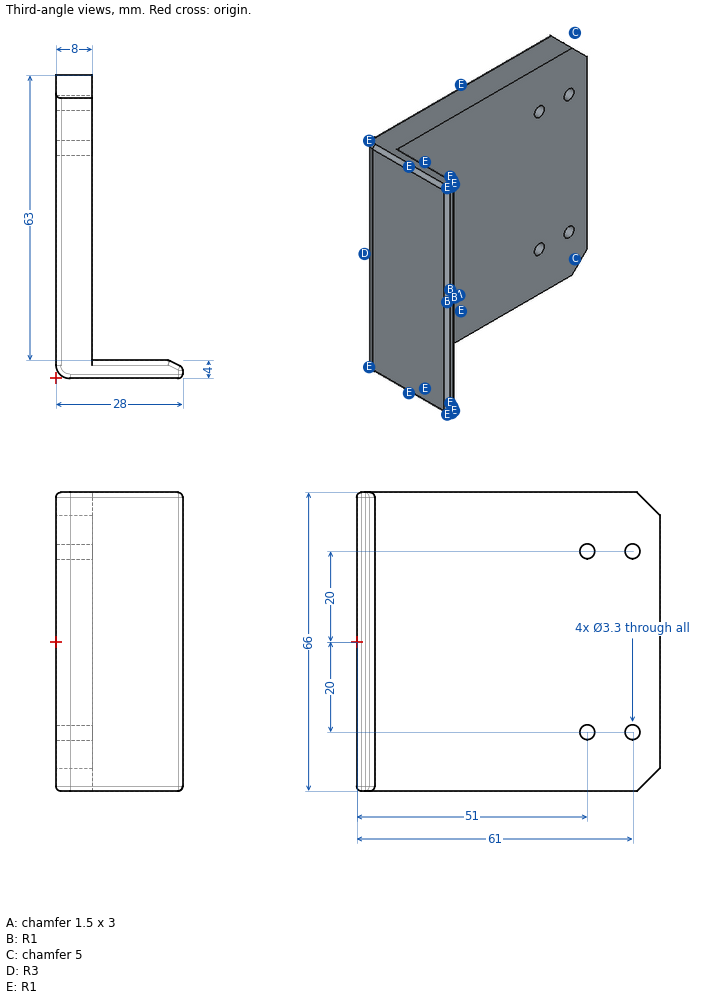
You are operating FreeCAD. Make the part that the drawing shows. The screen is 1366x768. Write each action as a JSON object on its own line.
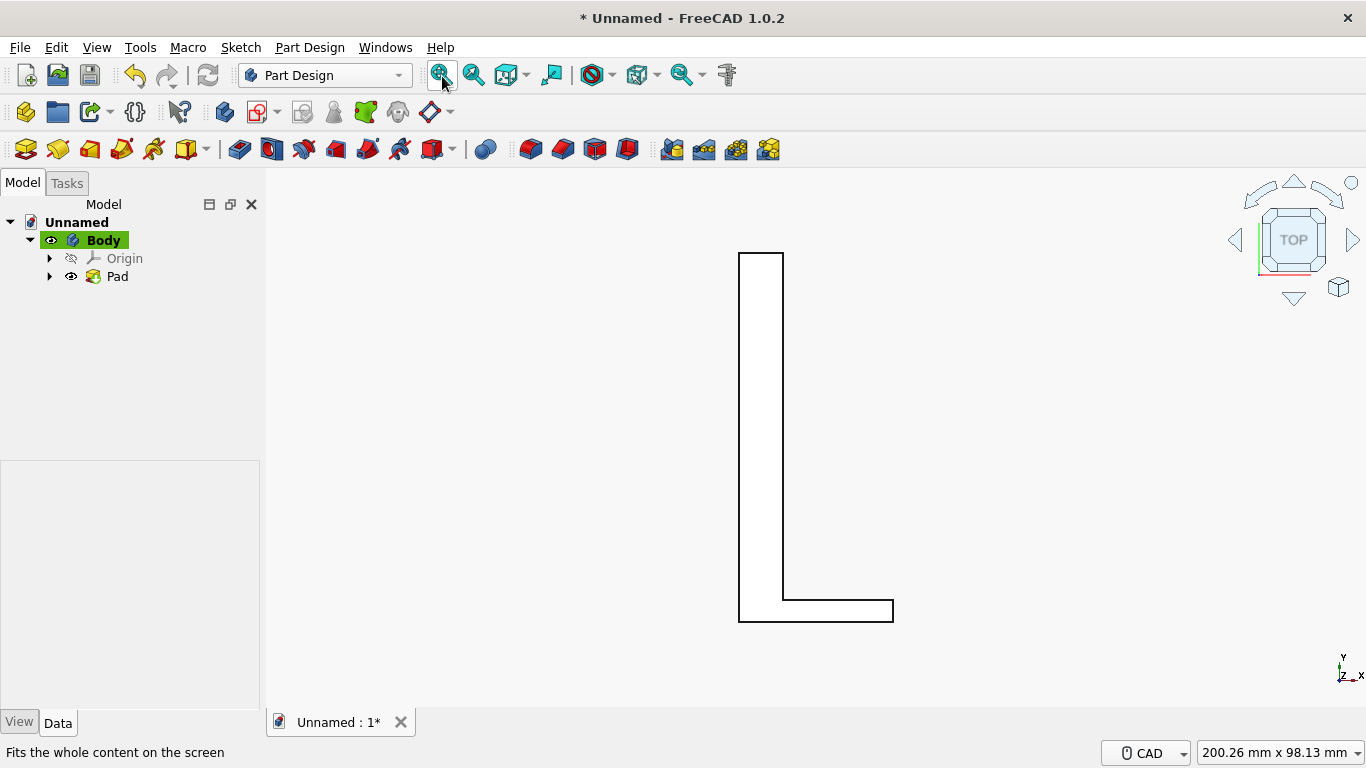
{"action": "key", "text": "1"}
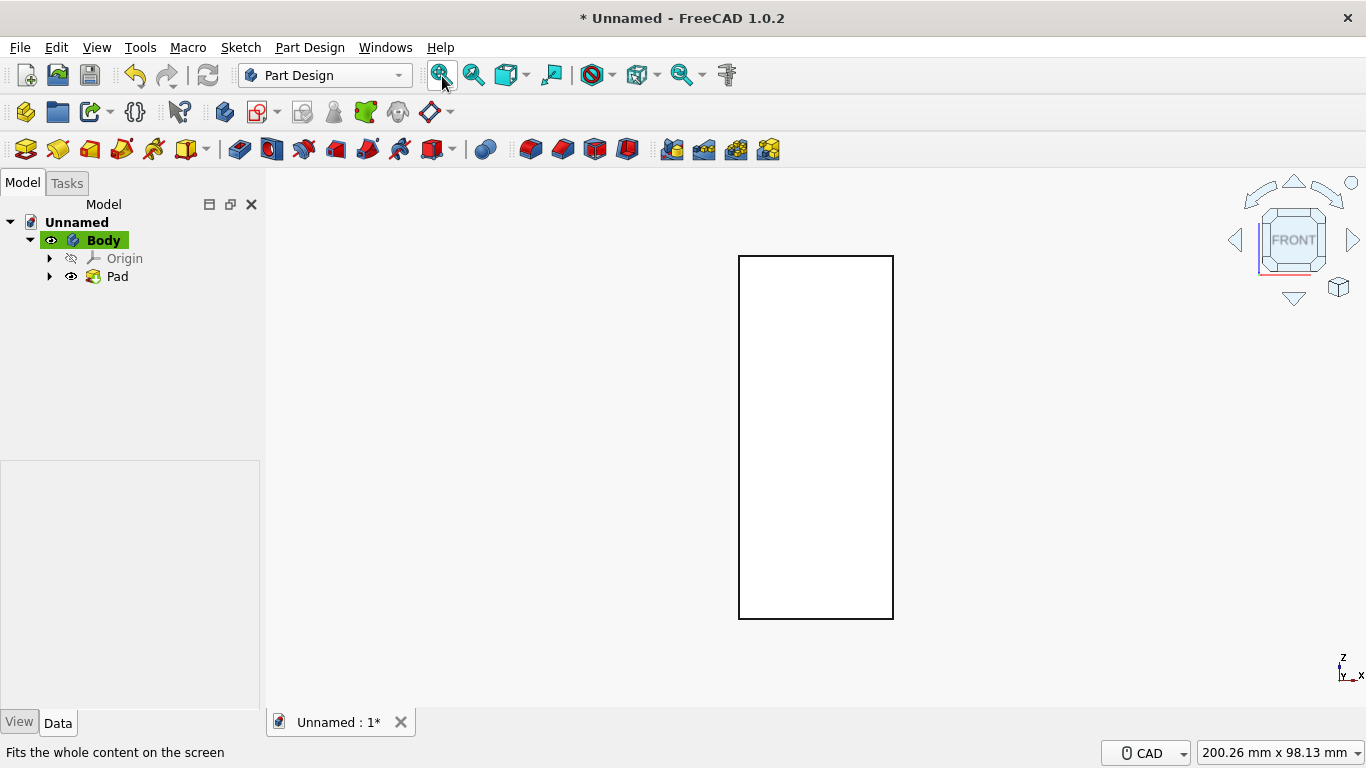
{"action": "key", "text": "3"}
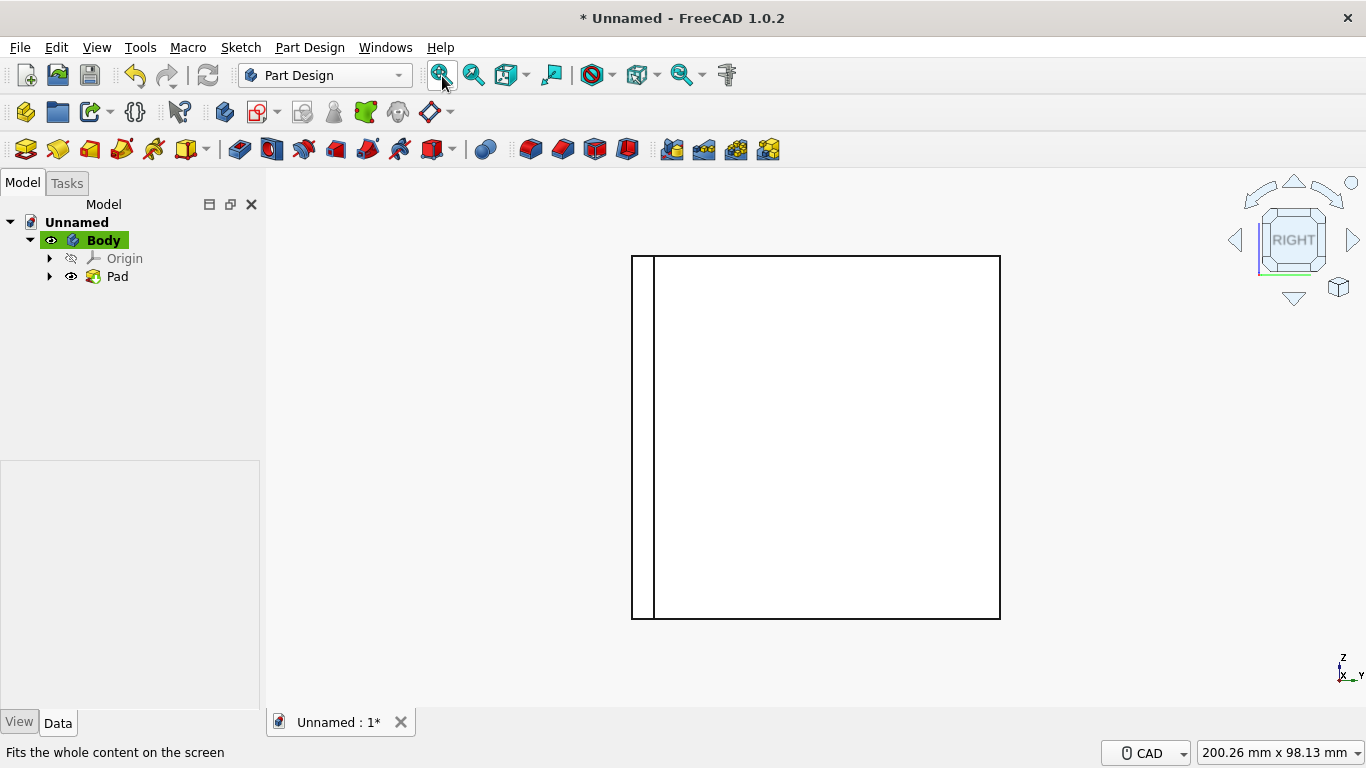
{"action": "left_click", "coordinate": [654, 436]}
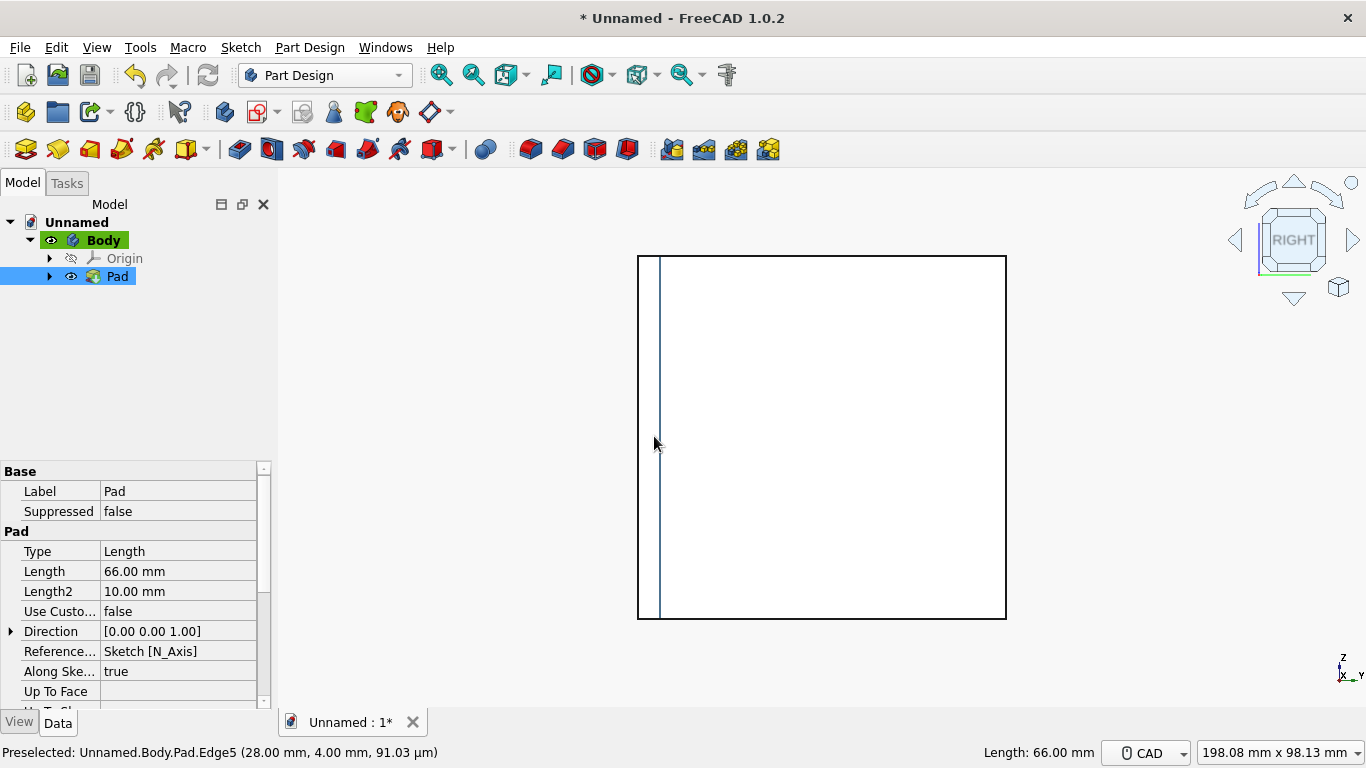
{"action": "left_click", "coordinate": [564, 150]}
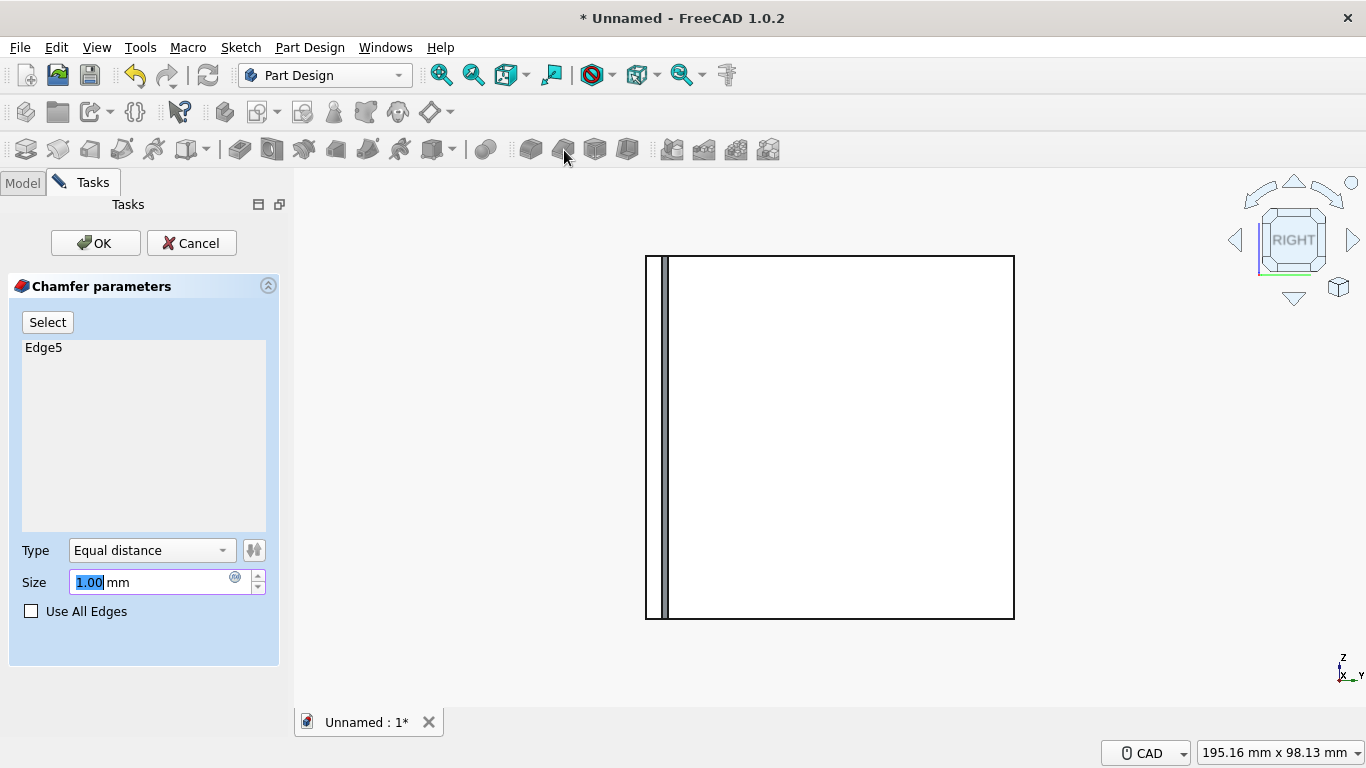
{"action": "type", "text": "1.5"}
{"action": "key", "text": "Tab"}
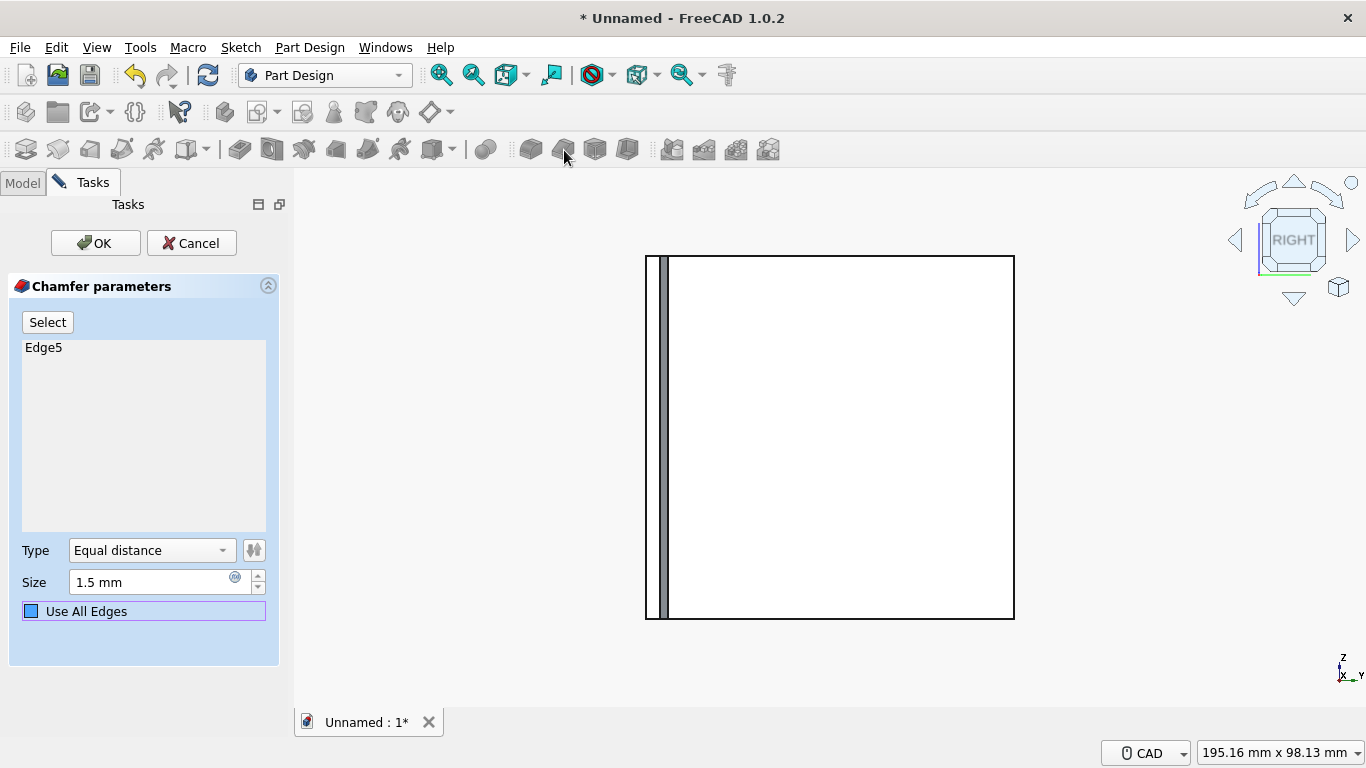
{"action": "left_click", "coordinate": [153, 550]}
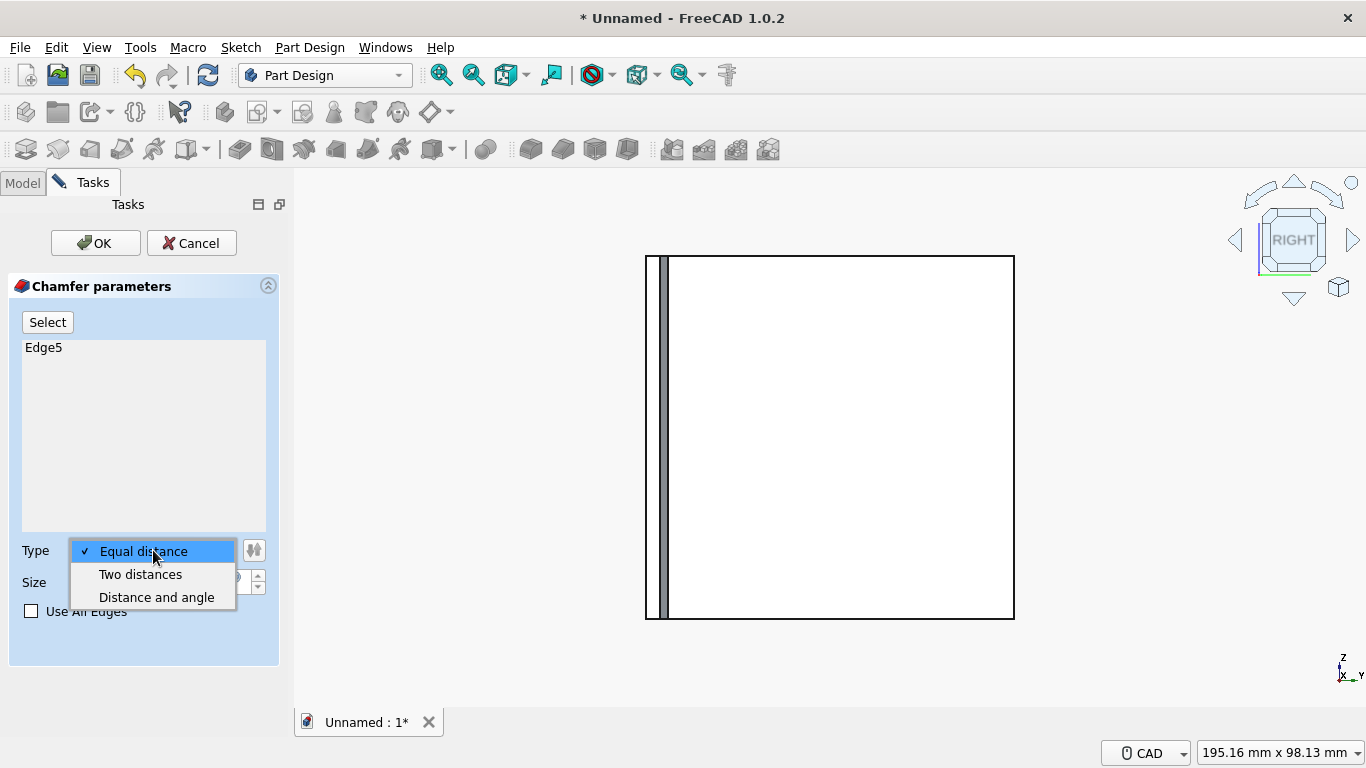
{"action": "left_click", "coordinate": [152, 574]}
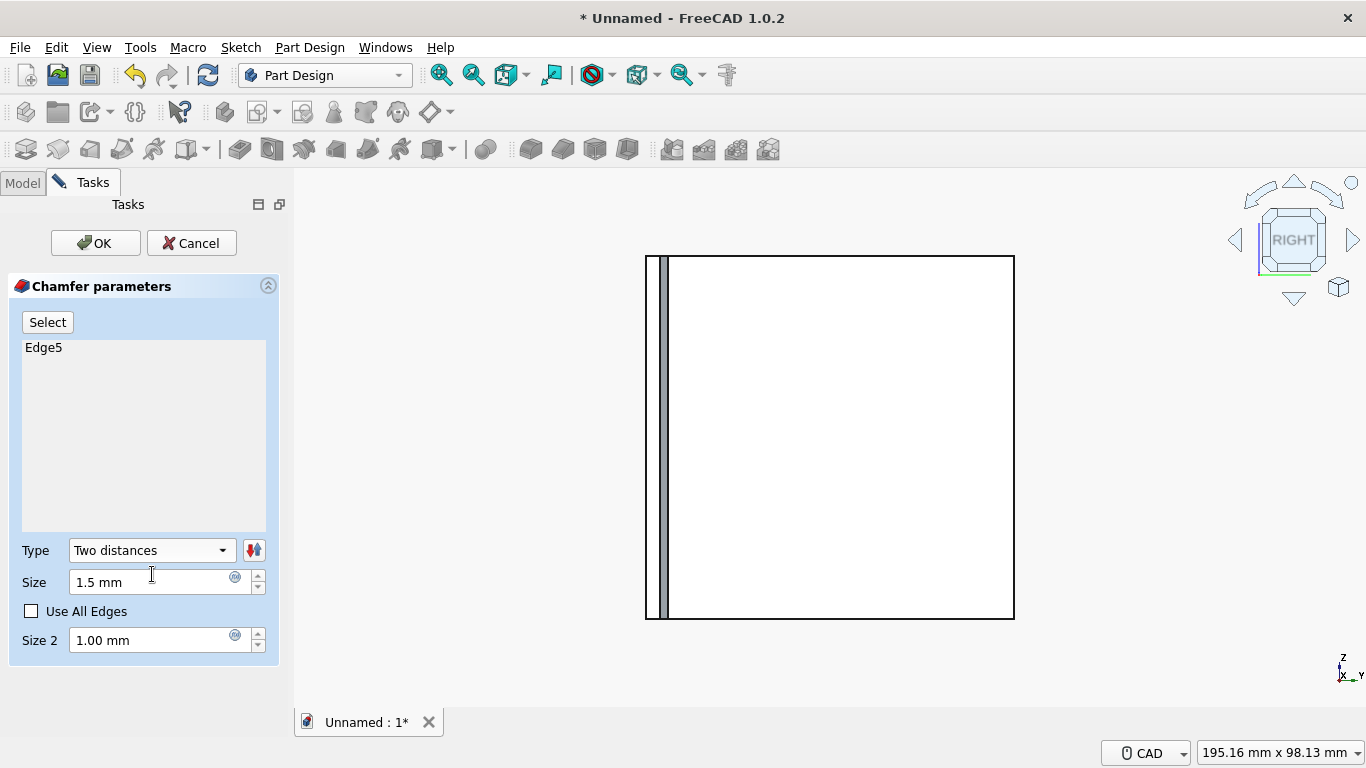
{"action": "triple_click", "coordinate": [160, 640]}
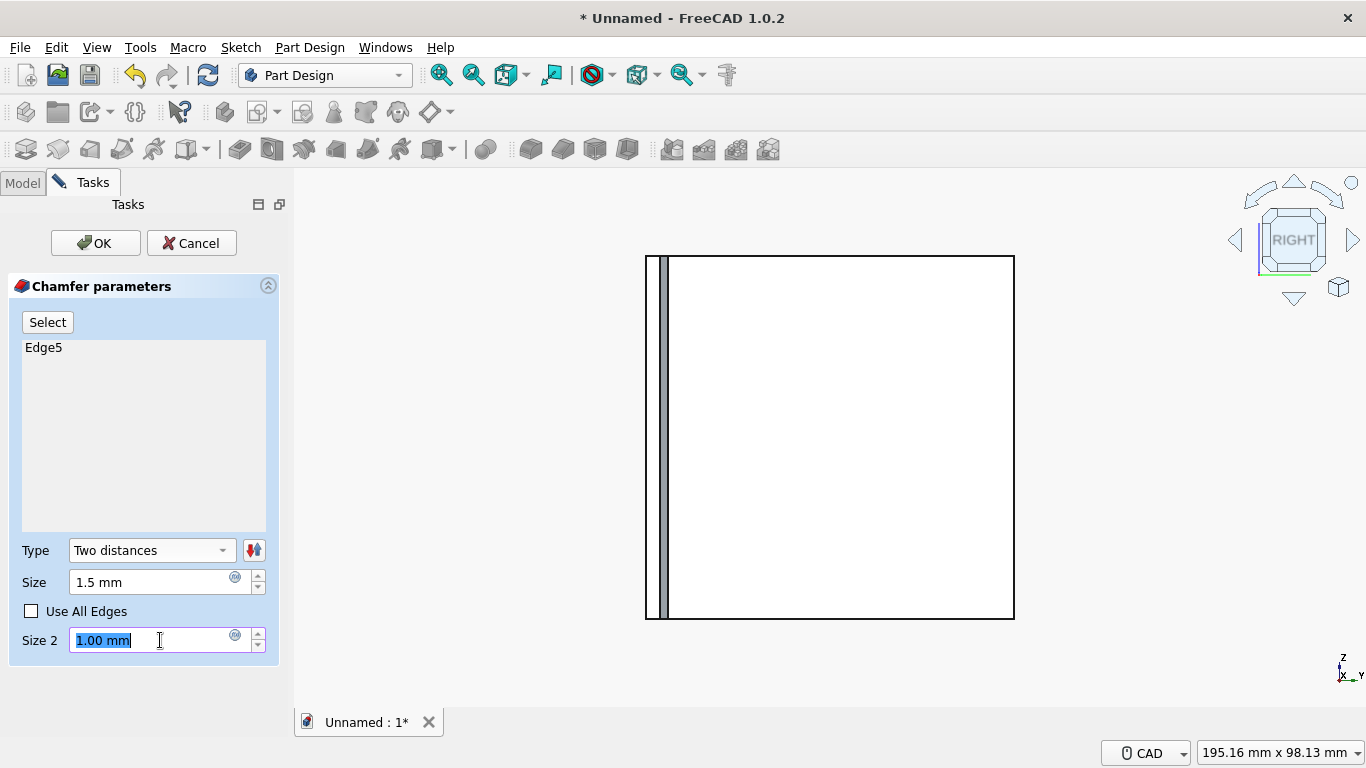
{"action": "type", "text": "3"}
{"action": "key", "text": "Tab"}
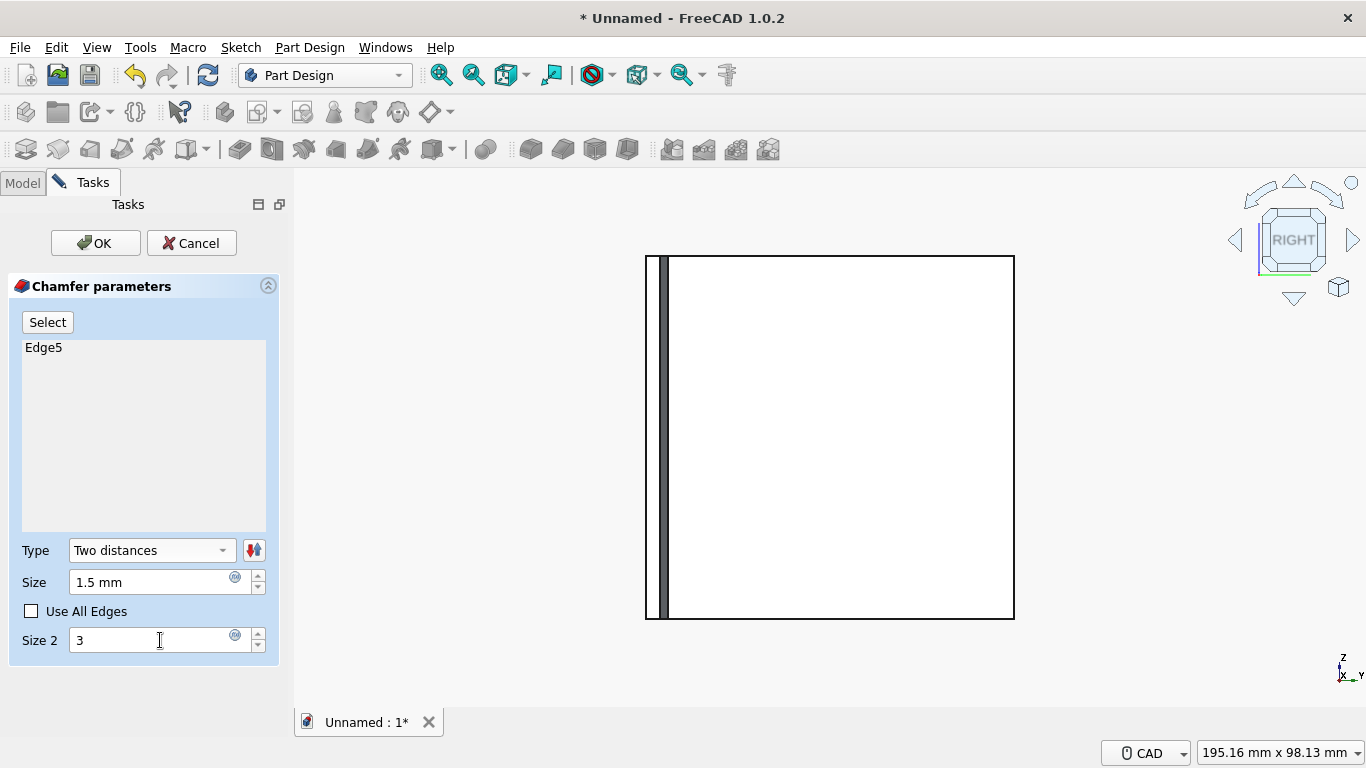
{"action": "left_click", "coordinate": [96, 243]}